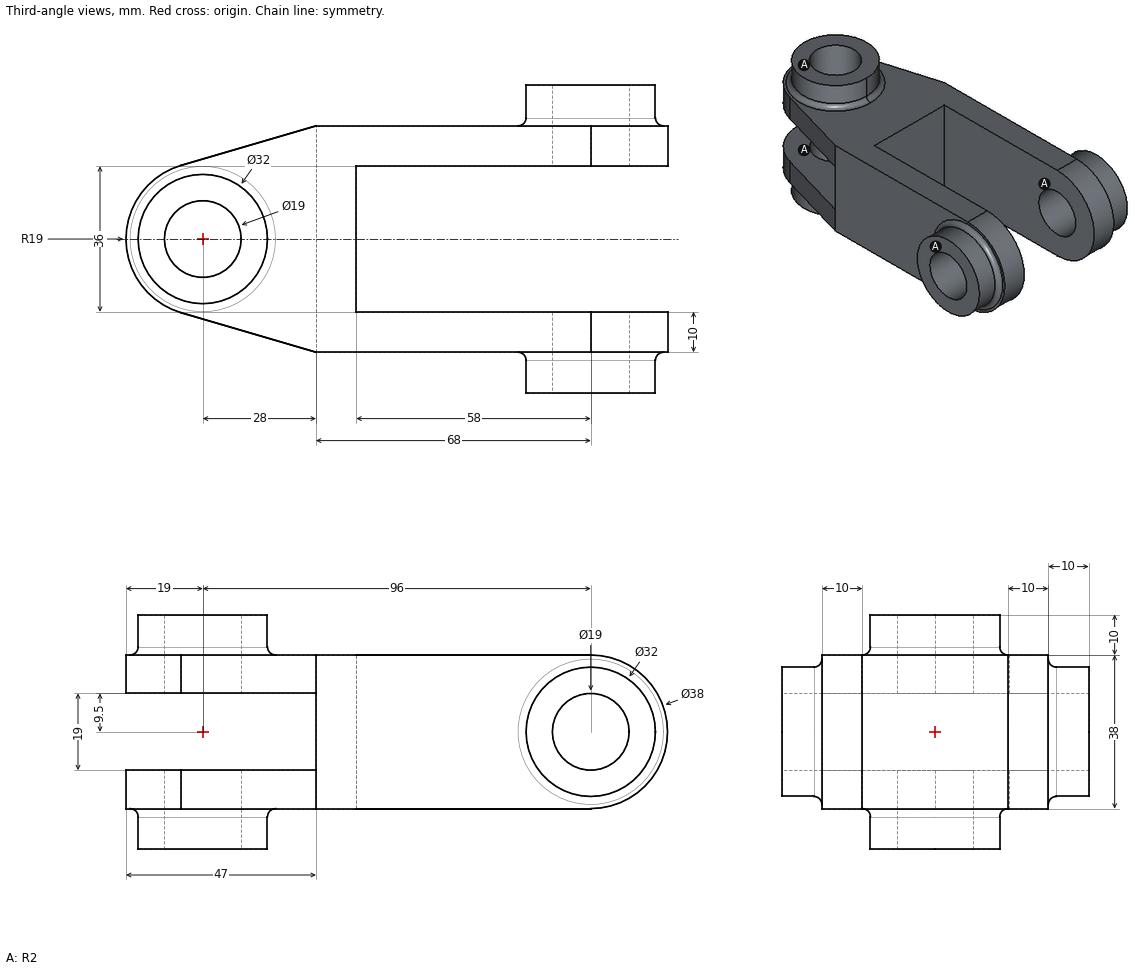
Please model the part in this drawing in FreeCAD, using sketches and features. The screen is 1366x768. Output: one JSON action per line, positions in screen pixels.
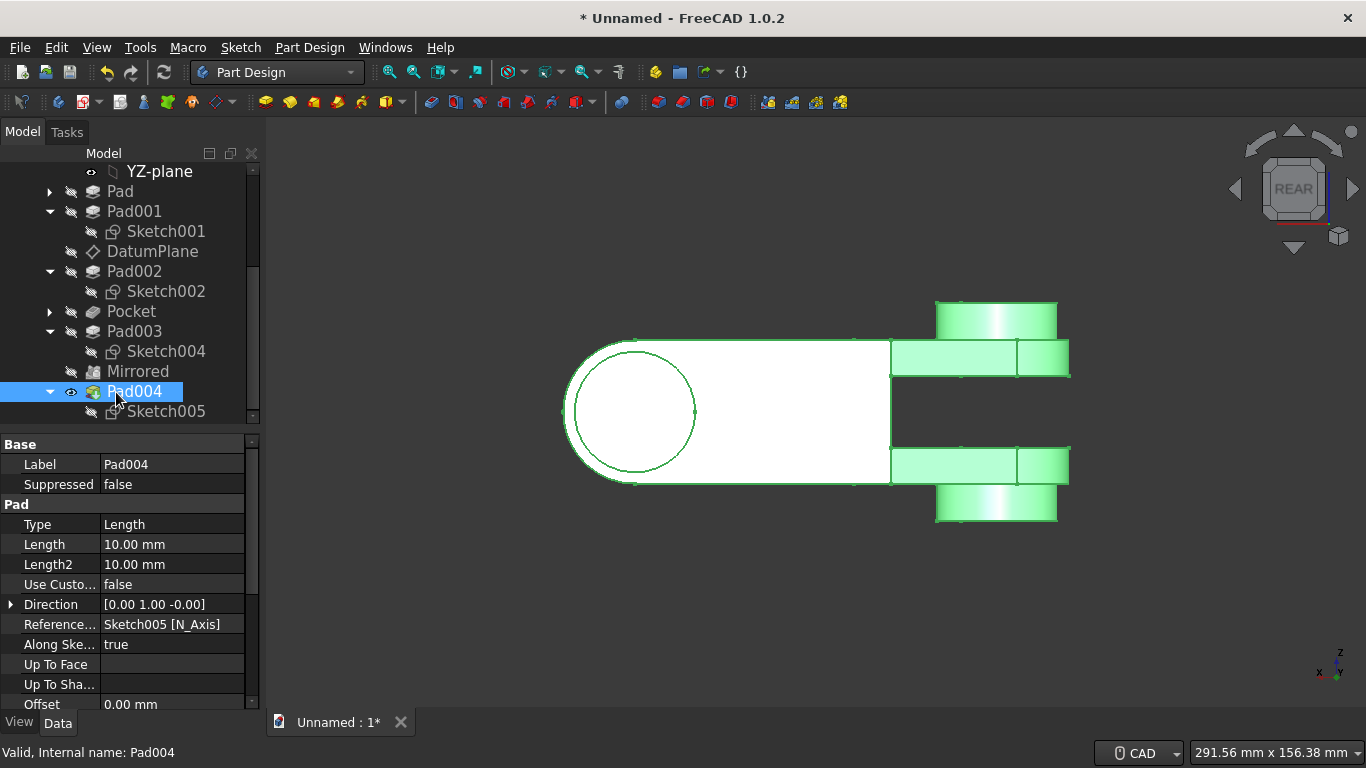
{"action": "left_click", "coordinate": [768, 102]}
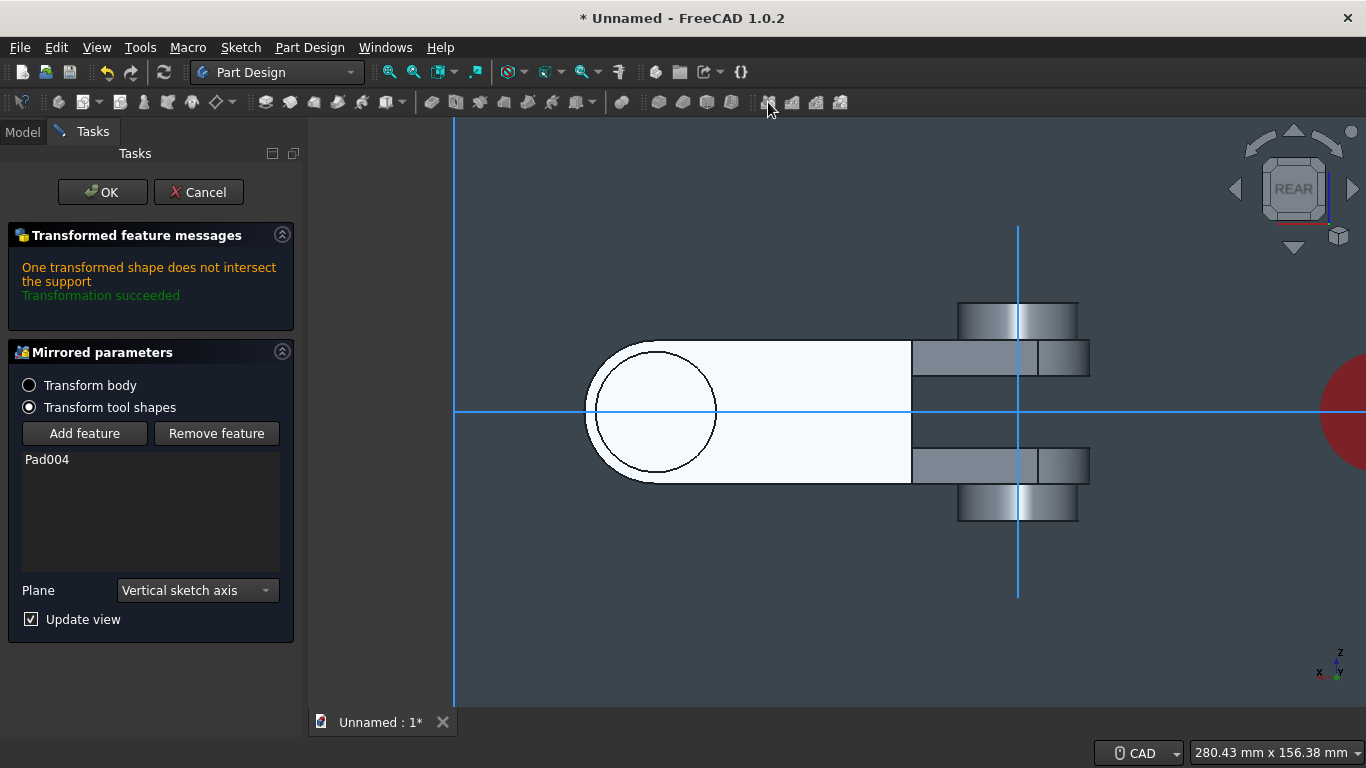
{"action": "left_click", "coordinate": [198, 590]}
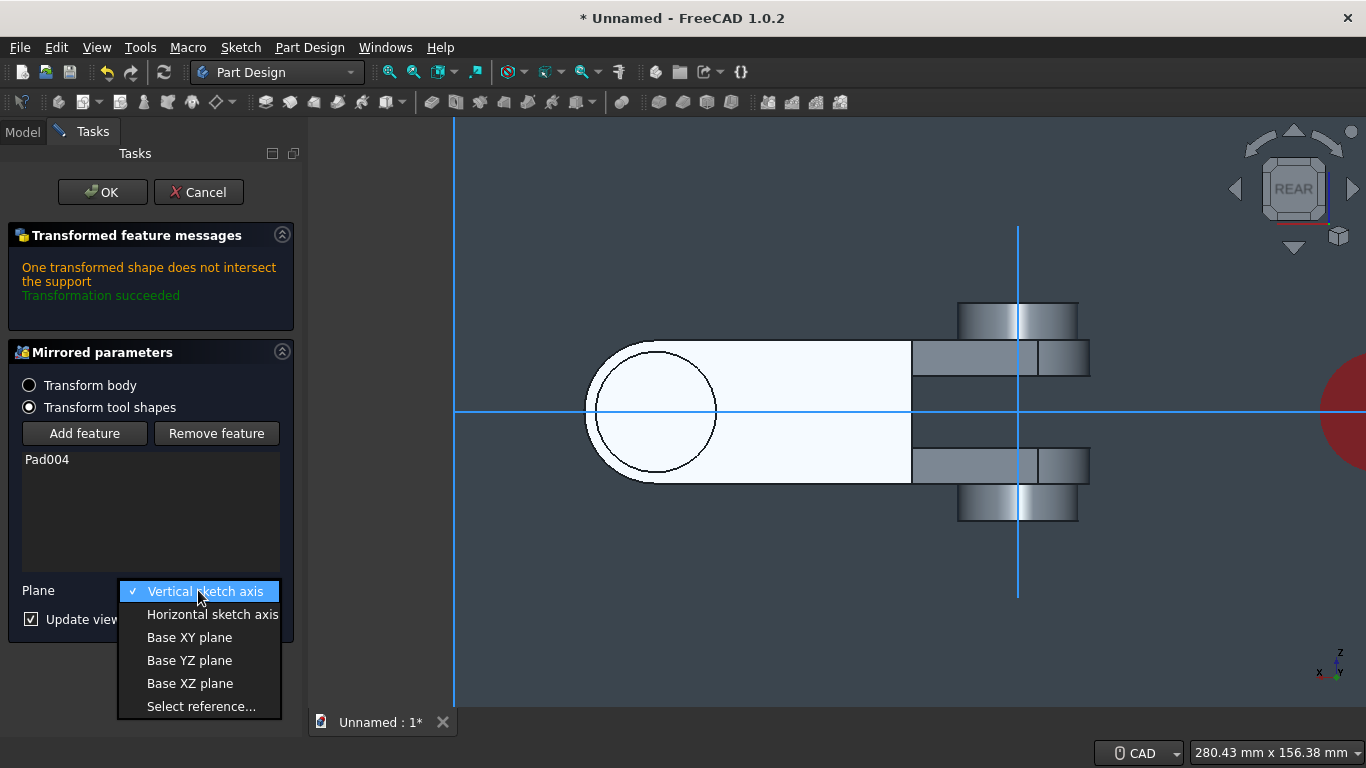
{"action": "left_click", "coordinate": [198, 684]}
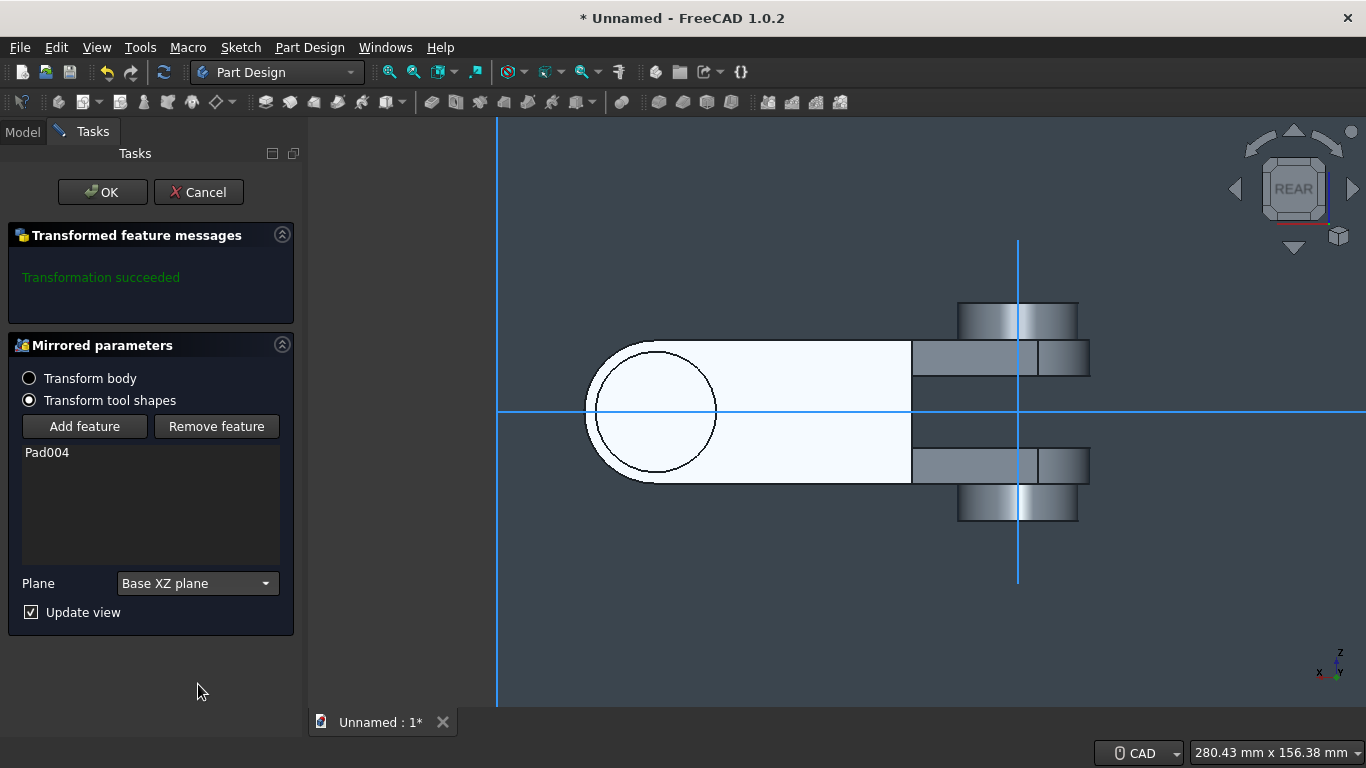
{"action": "left_click", "coordinate": [103, 192]}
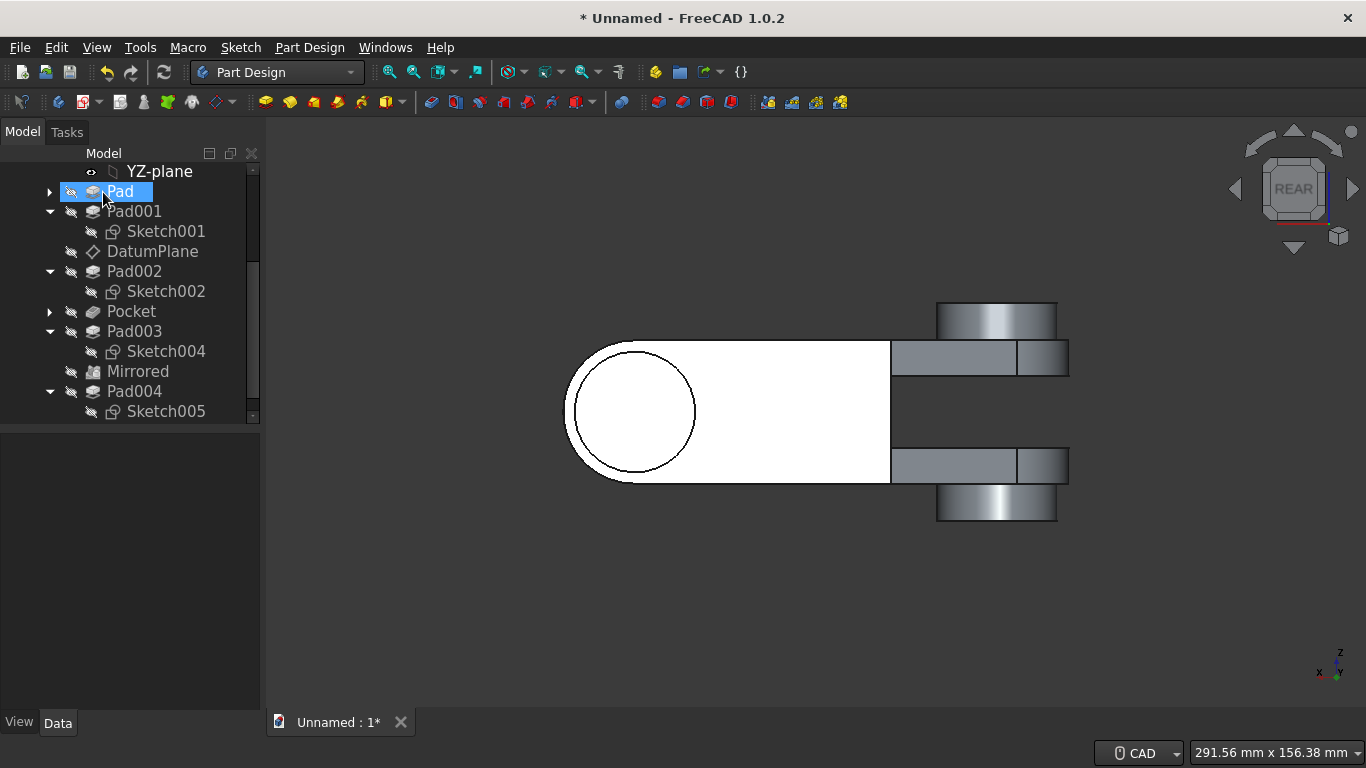
{"action": "key", "text": "0"}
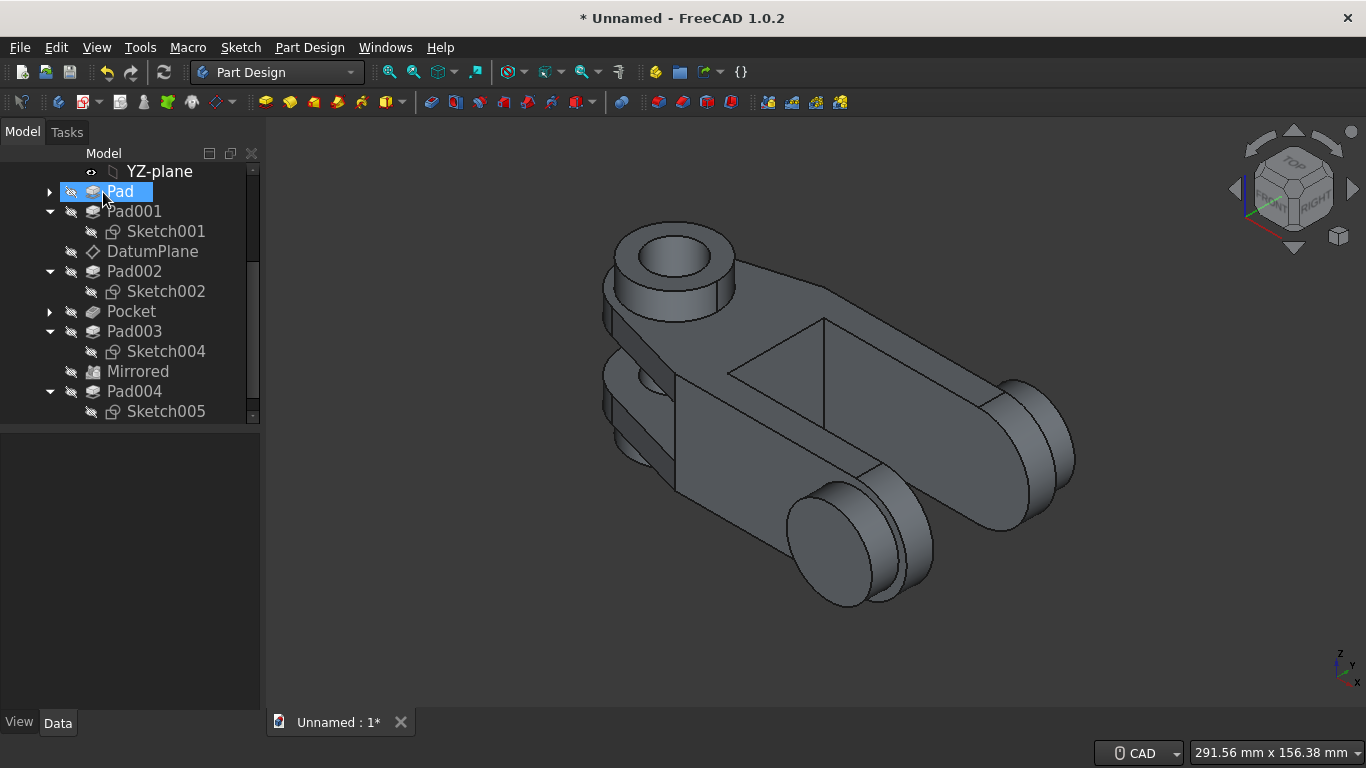
{"action": "left_click", "coordinate": [829, 551]}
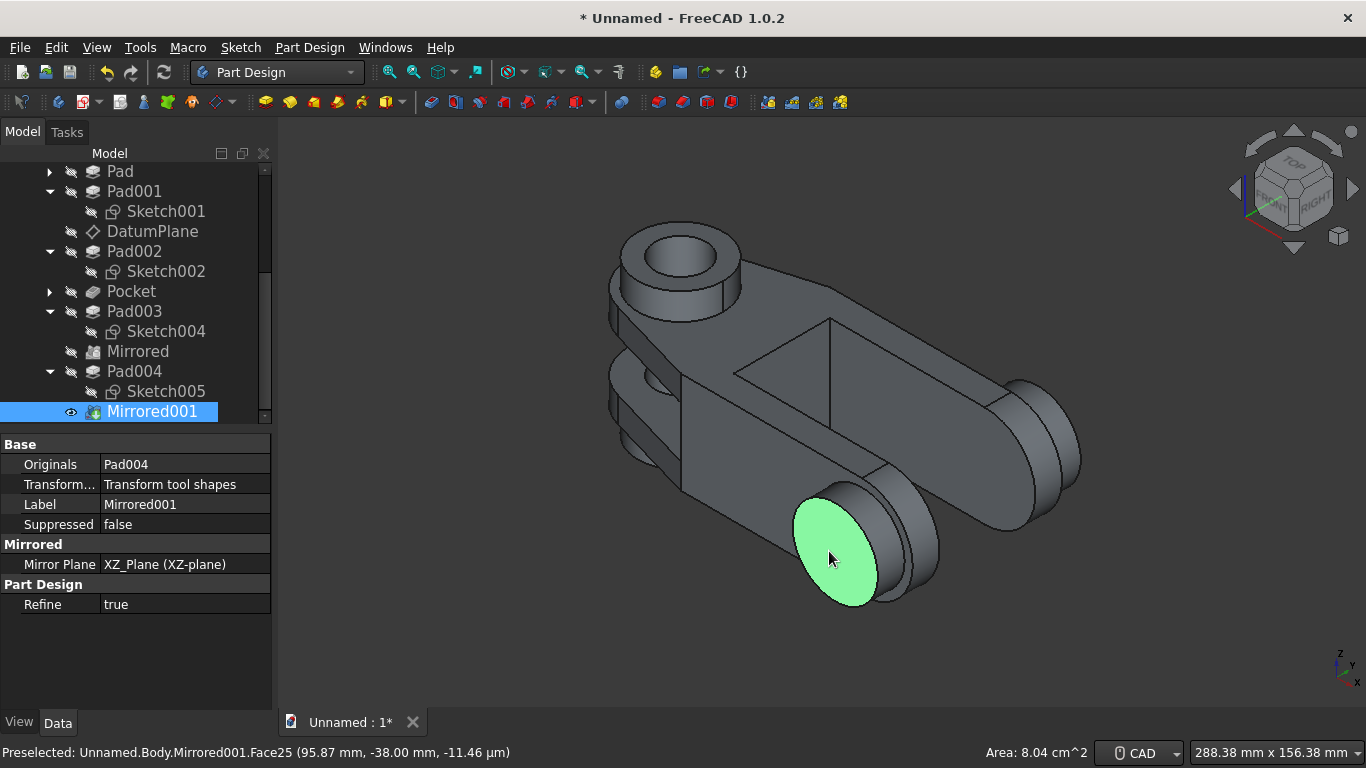
{"action": "left_click", "coordinate": [84, 102]}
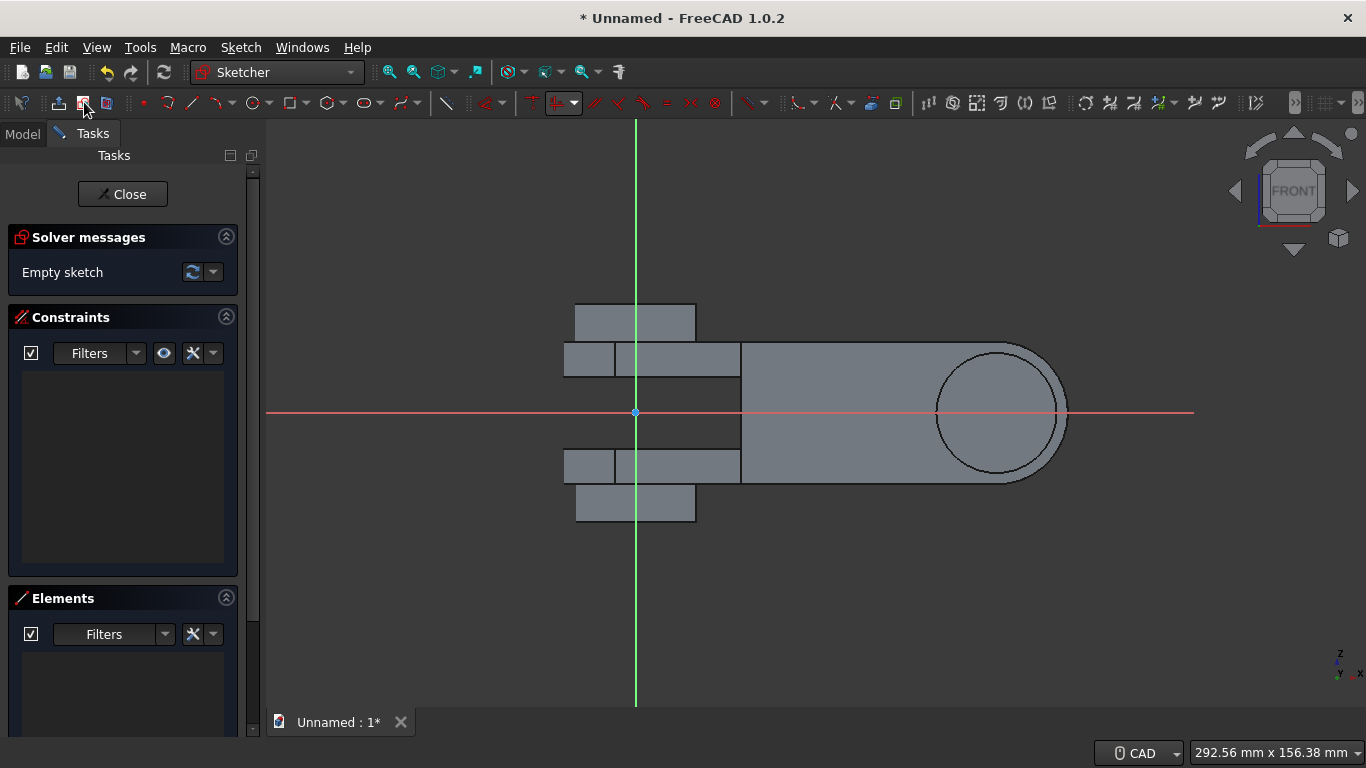
{"action": "scroll", "coordinate": [1059, 413], "scroll_direction": "up", "scroll_amount": 8}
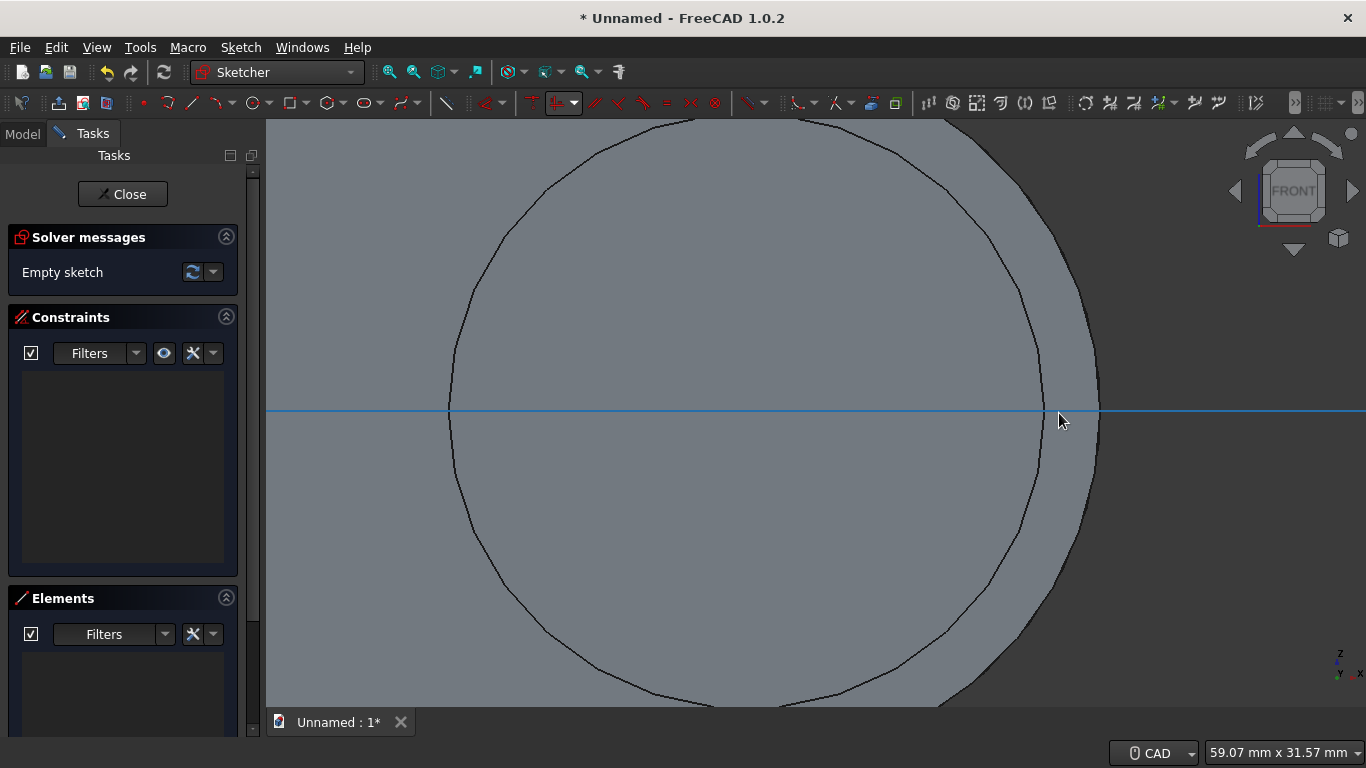
{"action": "left_click", "coordinate": [254, 104]}